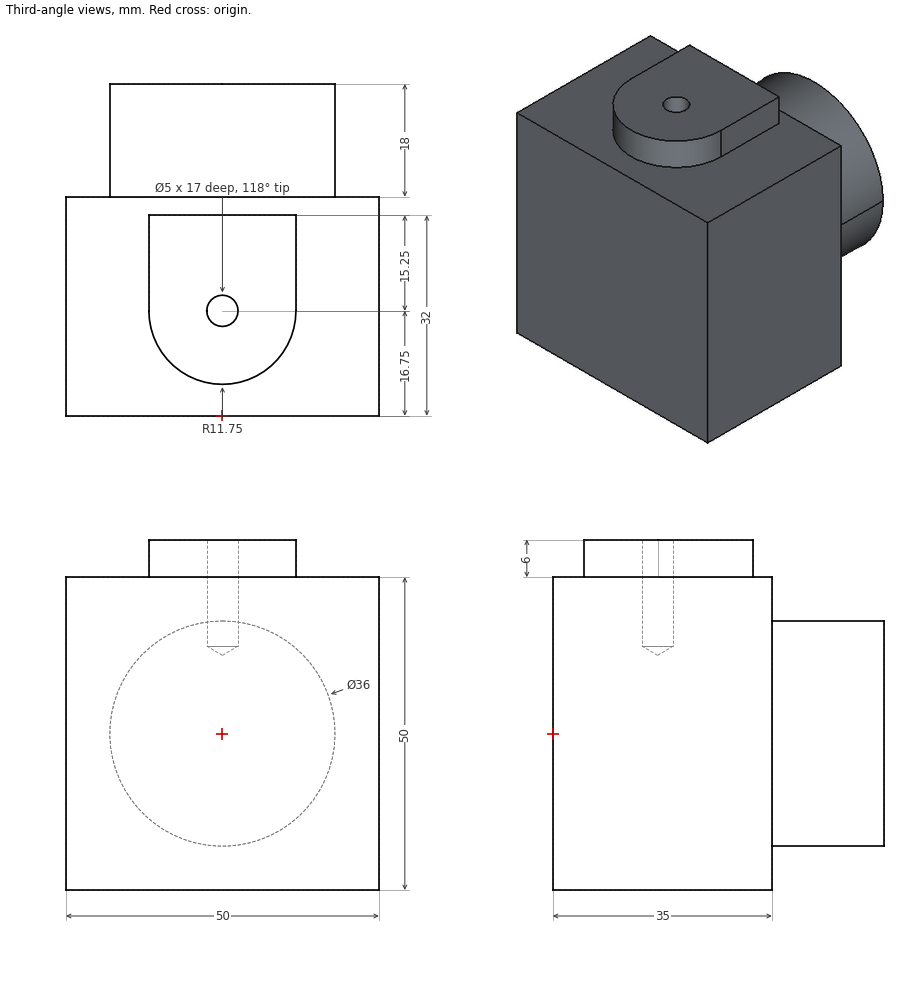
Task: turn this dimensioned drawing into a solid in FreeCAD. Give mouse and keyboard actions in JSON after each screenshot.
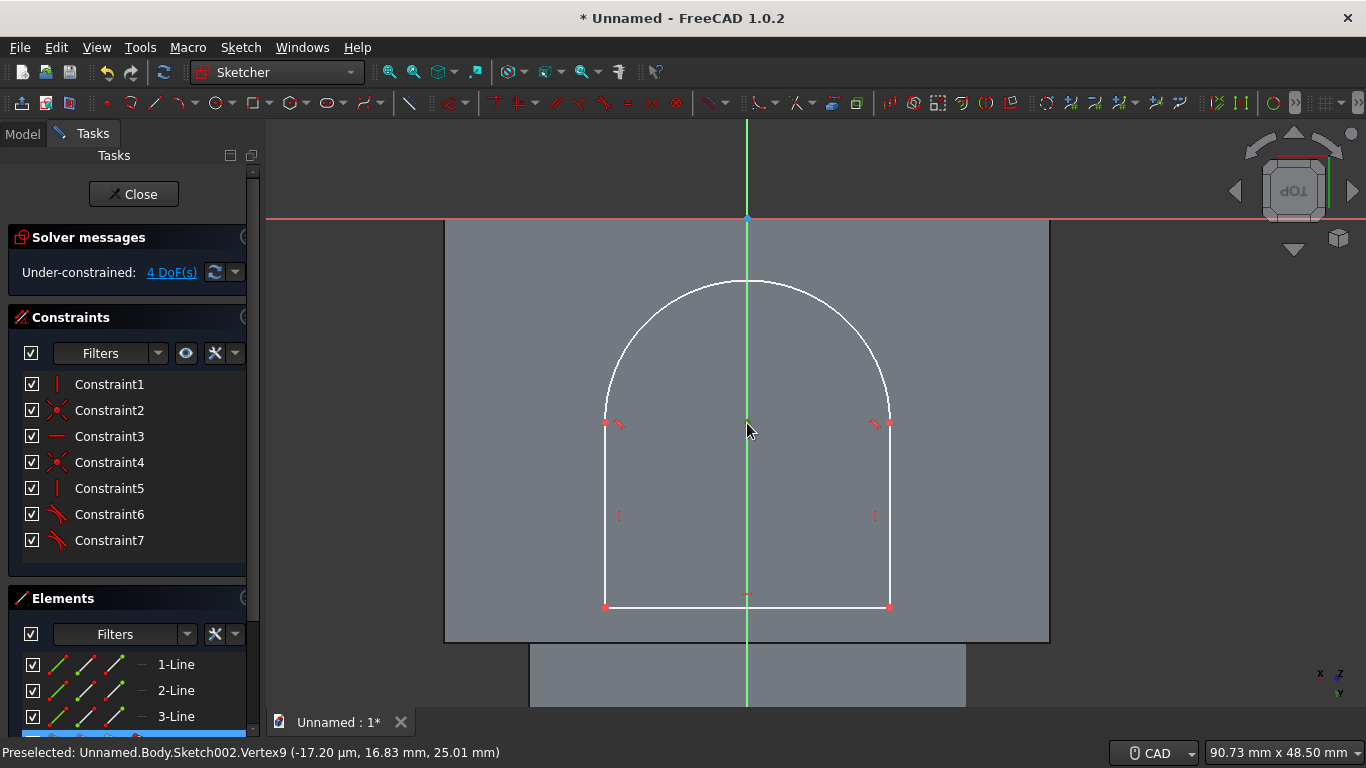
{"action": "left_click", "coordinate": [747, 641]}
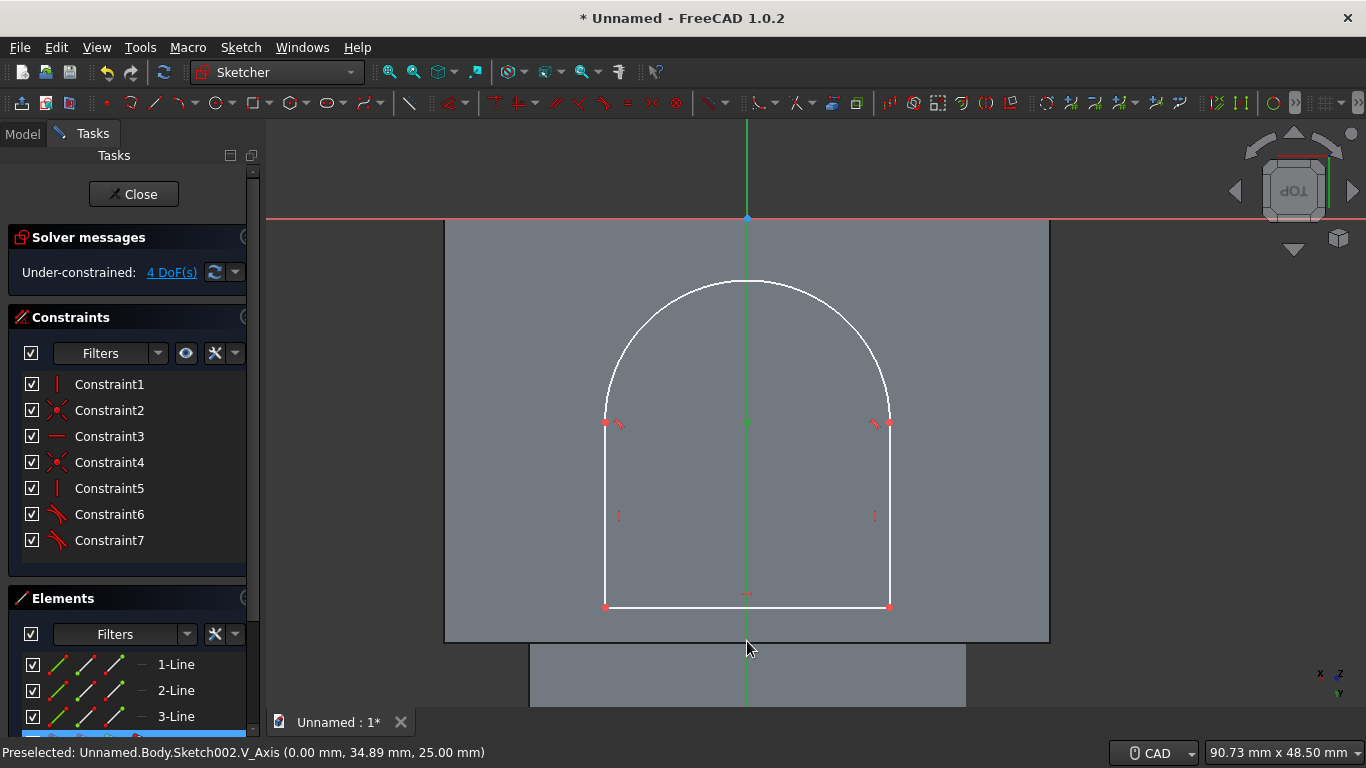
{"action": "key", "text": "c"}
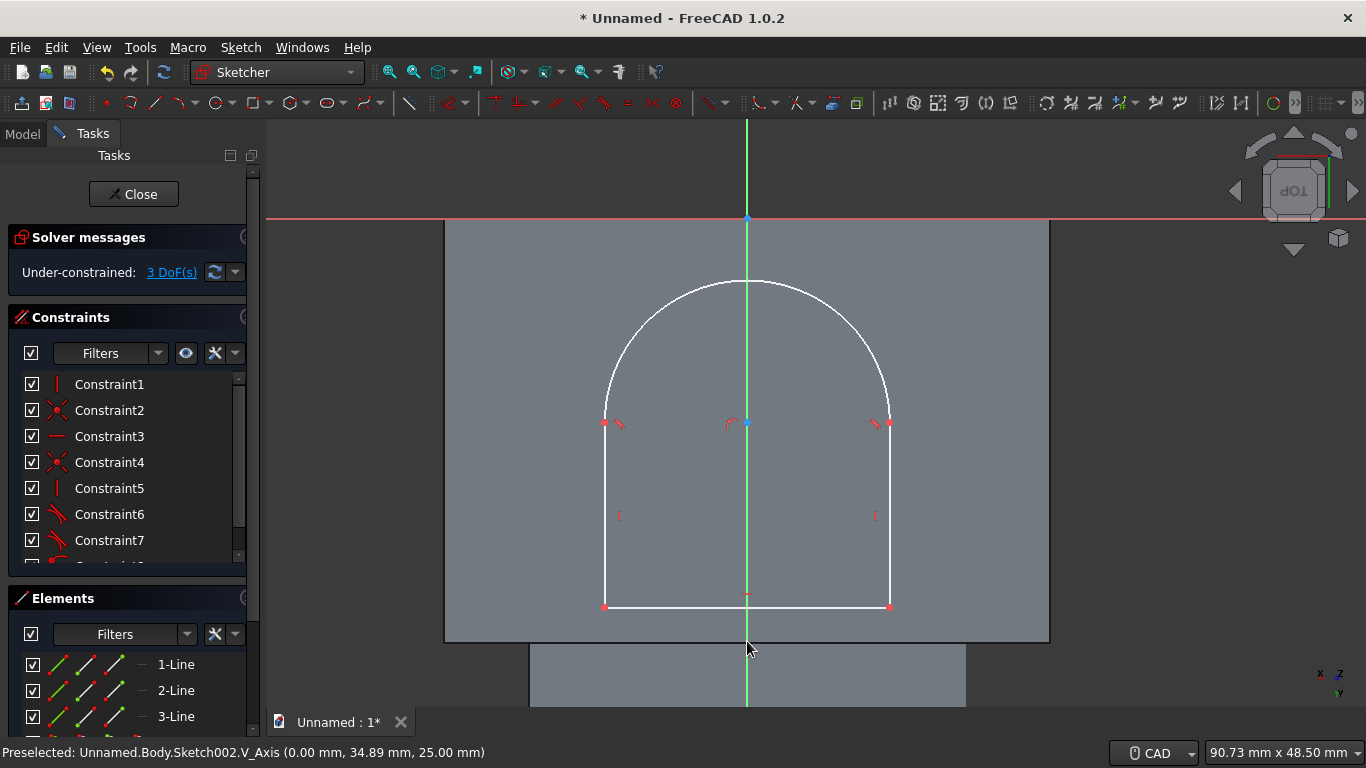
{"action": "key", "text": "d"}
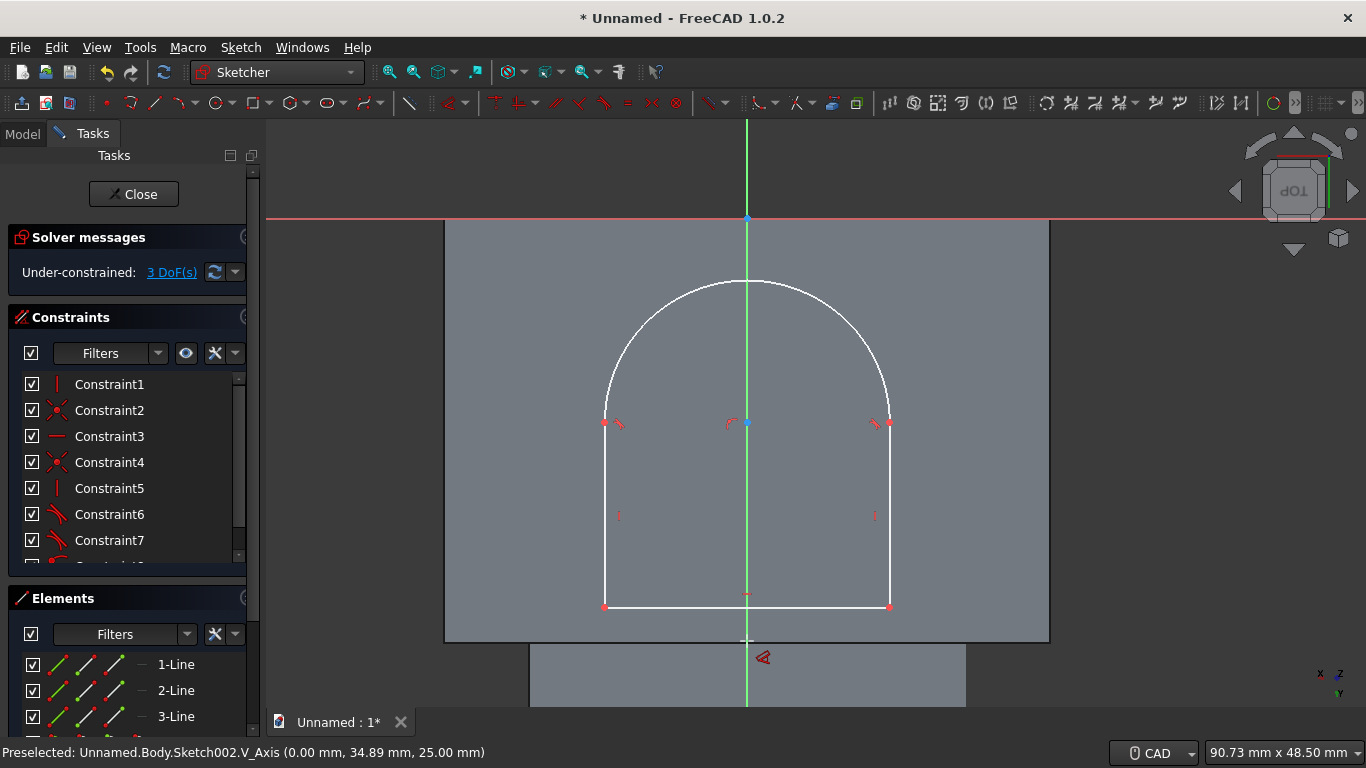
{"action": "left_click", "coordinate": [831, 308]}
{"action": "left_click", "coordinate": [850, 282]}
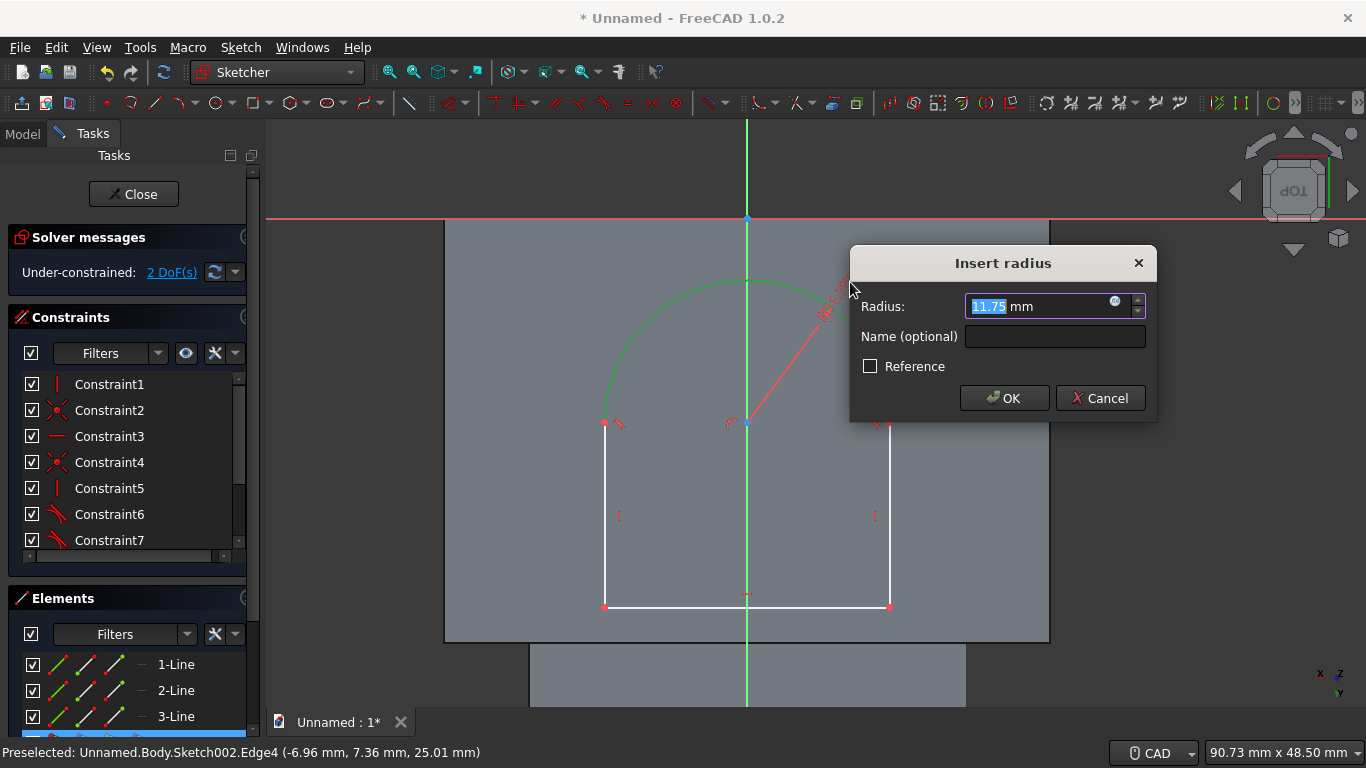
{"action": "type", "text": "11.75"}
{"action": "key", "text": "Return"}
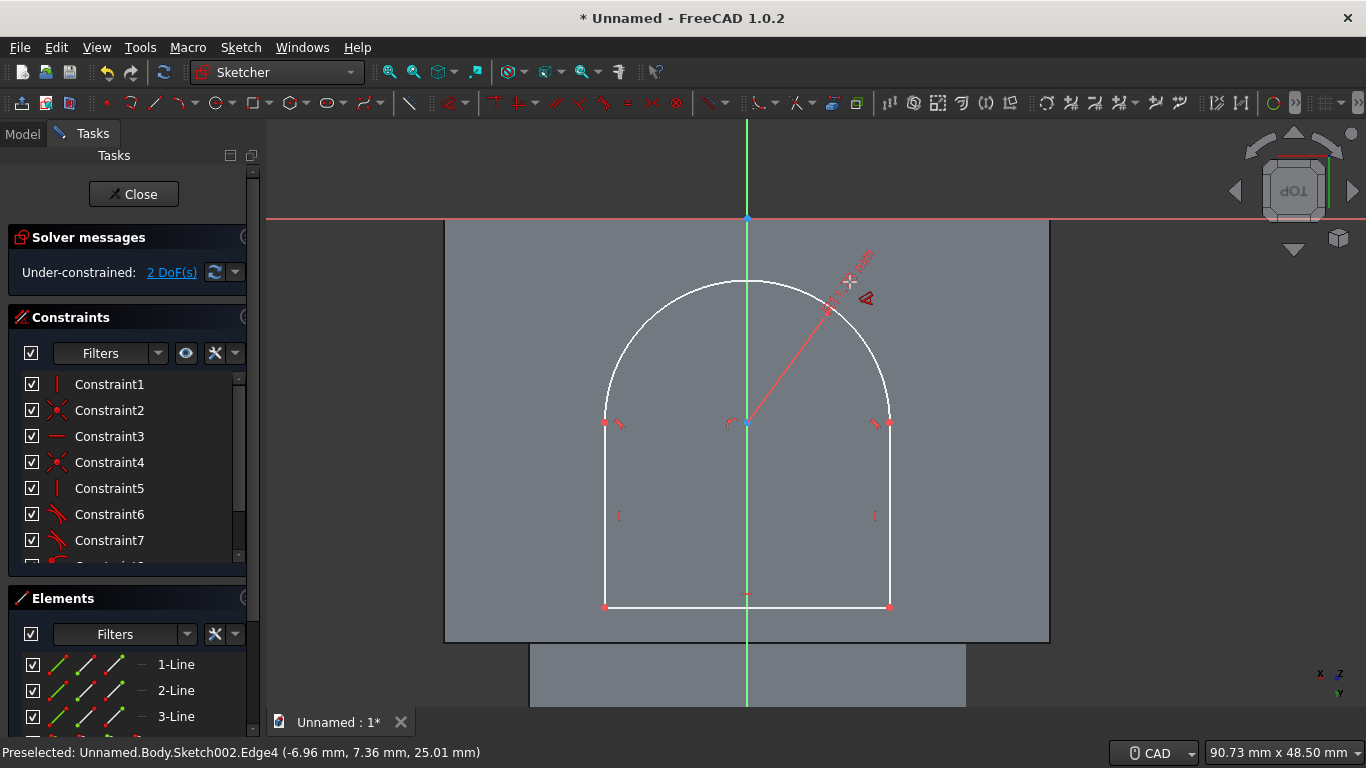
{"action": "left_click", "coordinate": [605, 608]}
{"action": "left_click", "coordinate": [571, 413]}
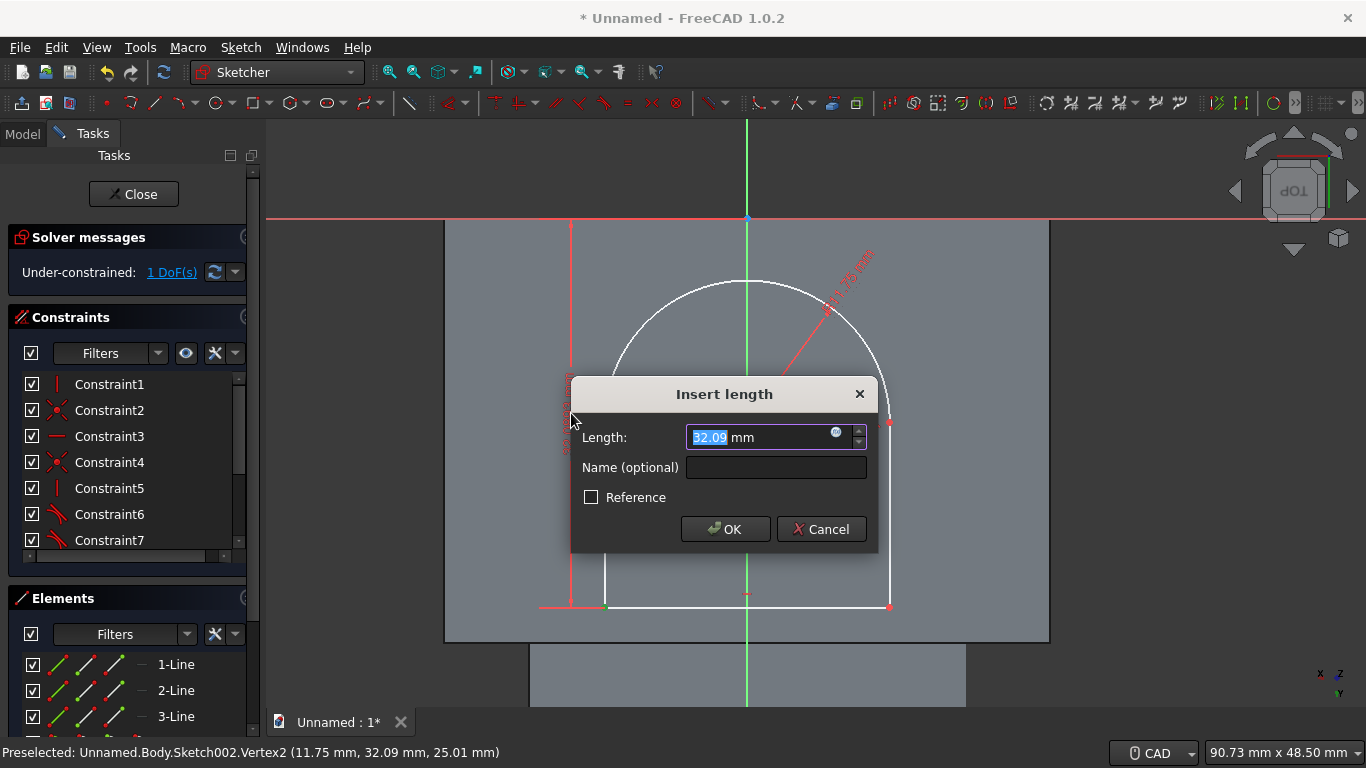
{"action": "type", "text": "32"}
{"action": "key", "text": "Return"}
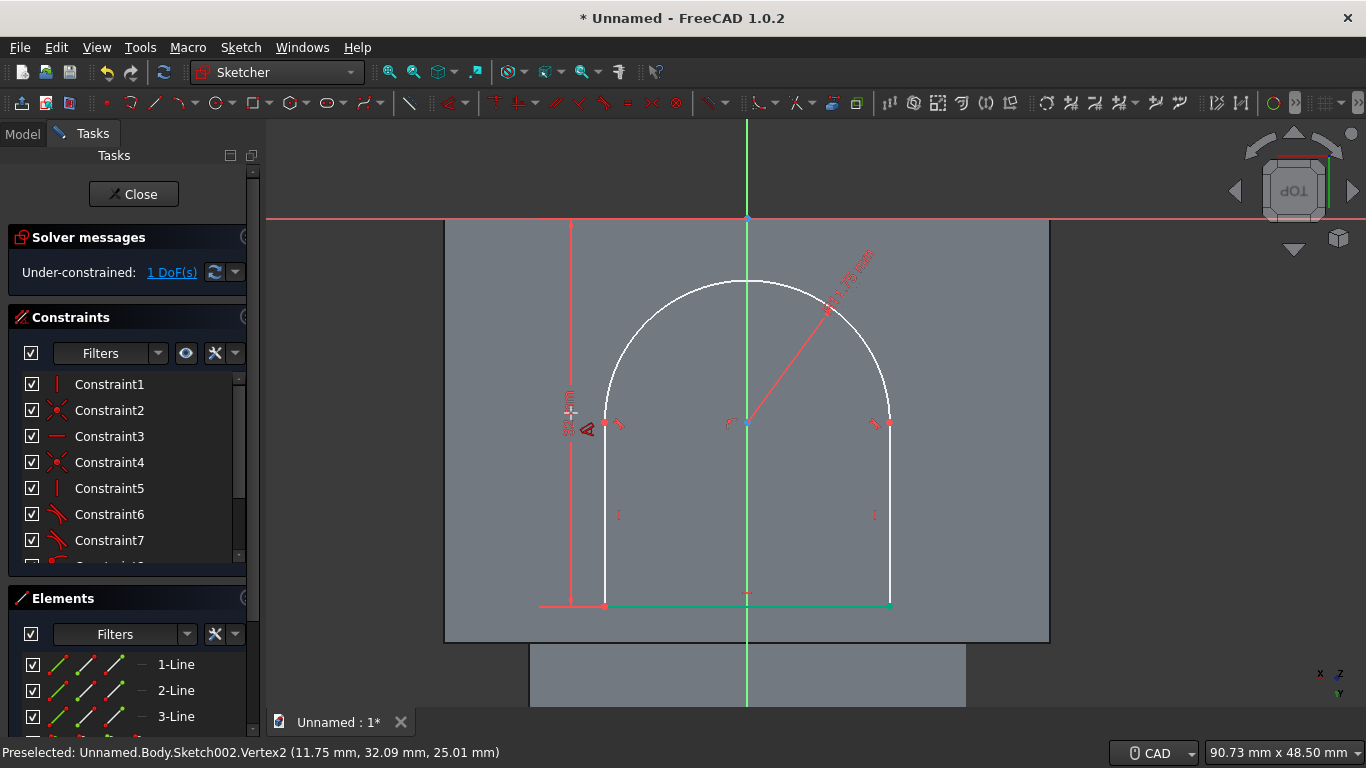
{"action": "left_click", "coordinate": [605, 478]}
{"action": "left_click", "coordinate": [571, 515]}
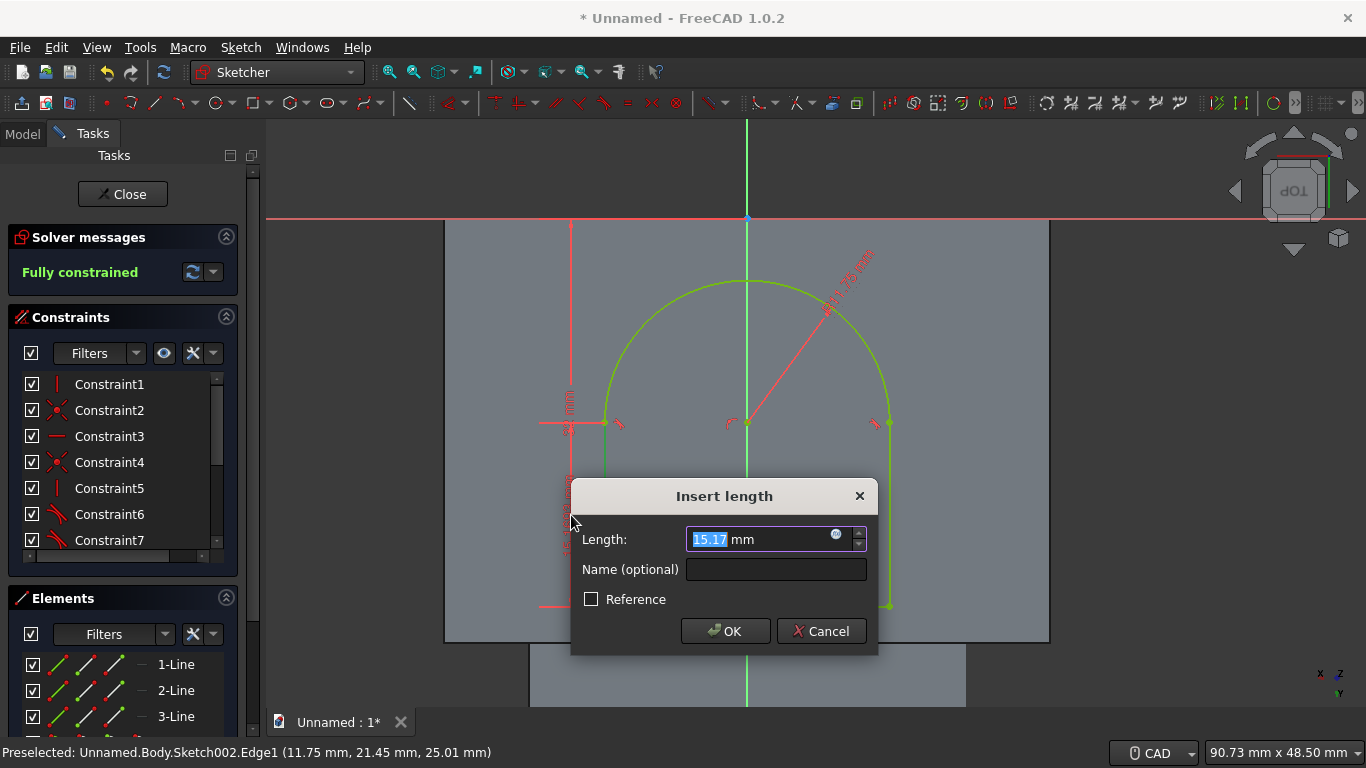
{"action": "type", "text": "15.25"}
{"action": "key", "text": "Return"}
{"action": "key", "text": "Escape"}